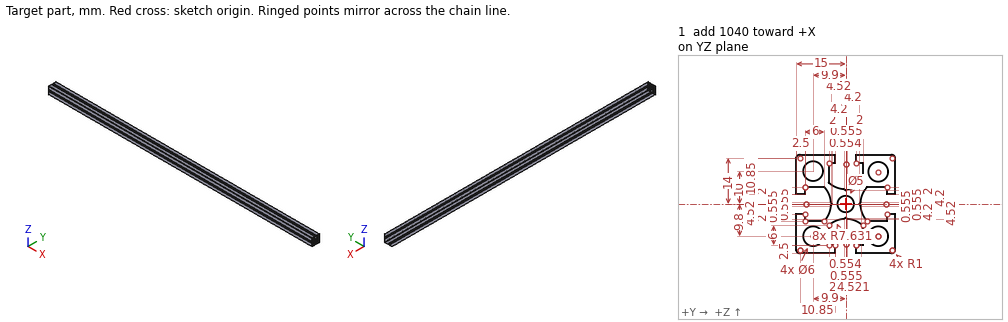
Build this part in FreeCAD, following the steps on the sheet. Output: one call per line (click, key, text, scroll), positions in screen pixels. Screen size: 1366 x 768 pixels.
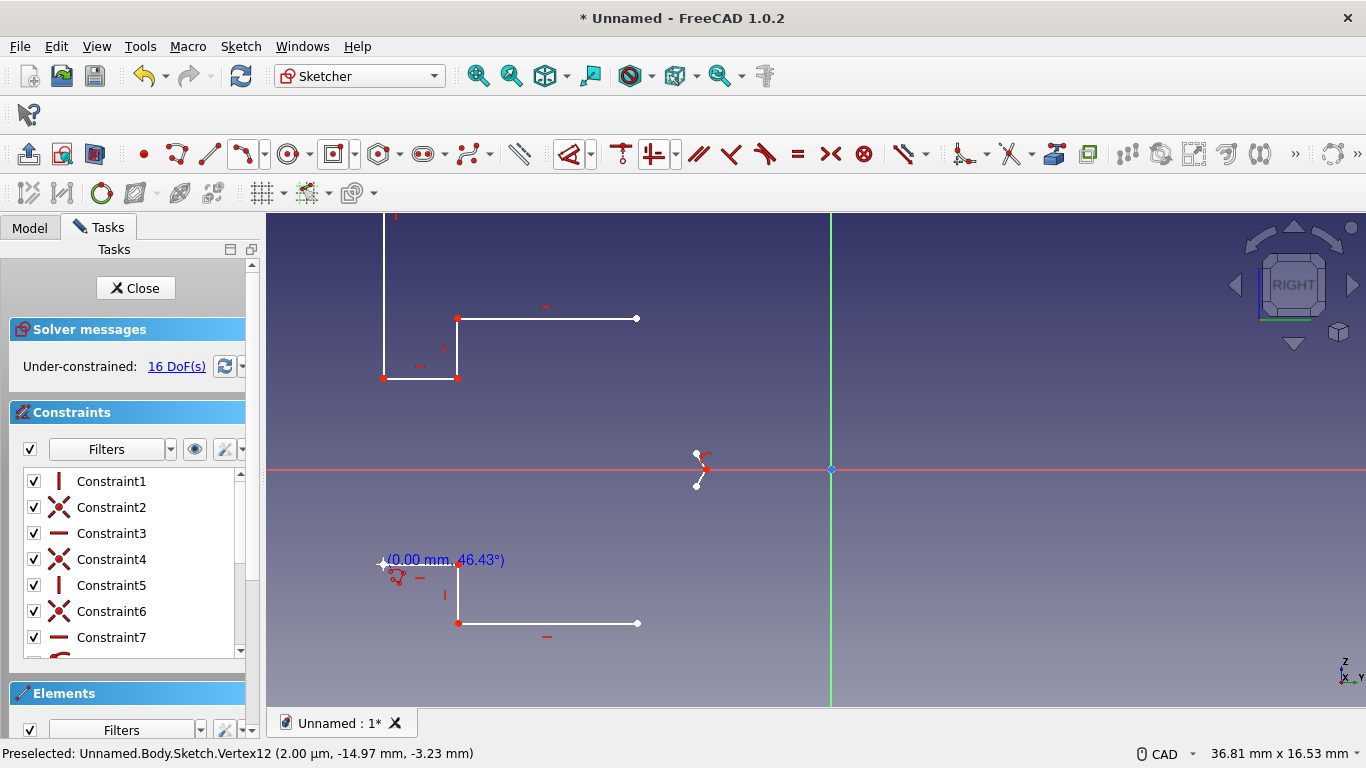
scroll(699, 454, down, 5)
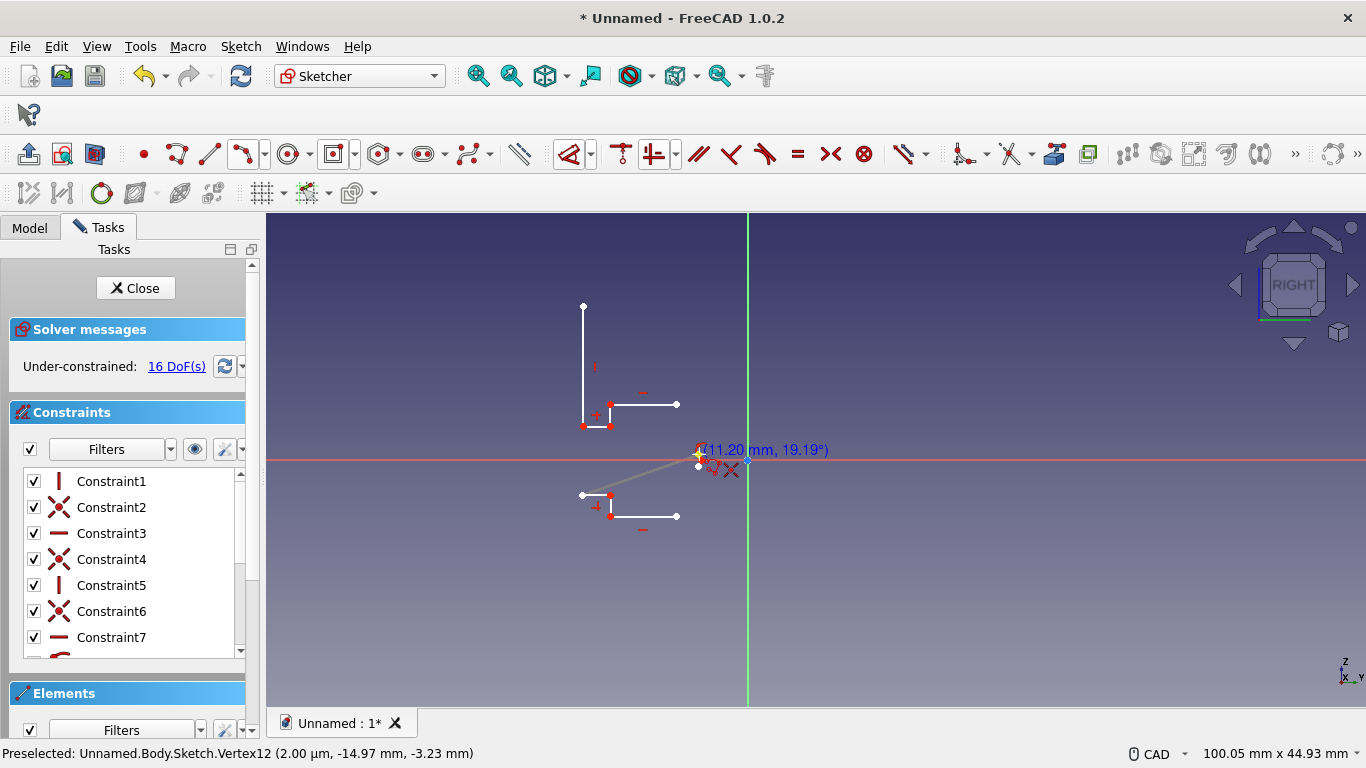
click(583, 614)
right_click(583, 614)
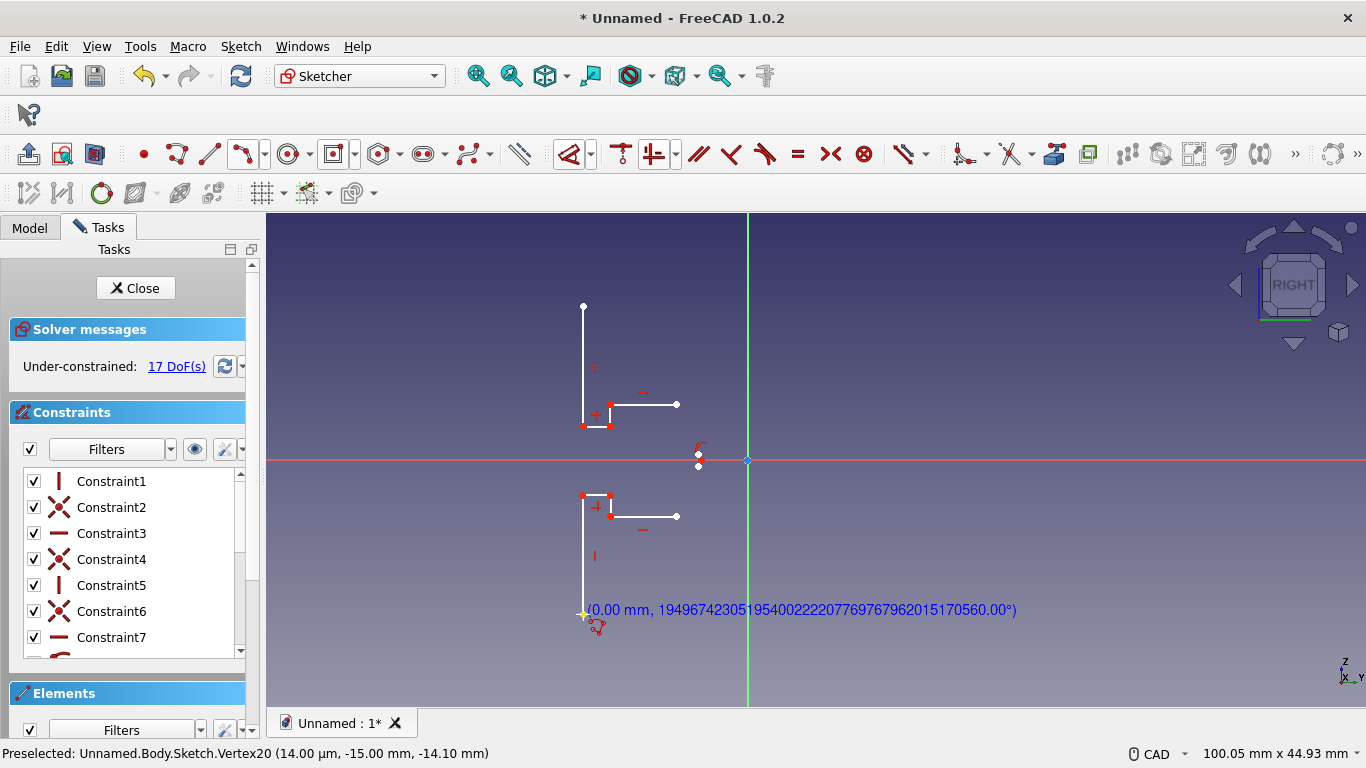
click(594, 625)
click(713, 625)
click(713, 597)
click(691, 597)
click(691, 531)
right_click(691, 531)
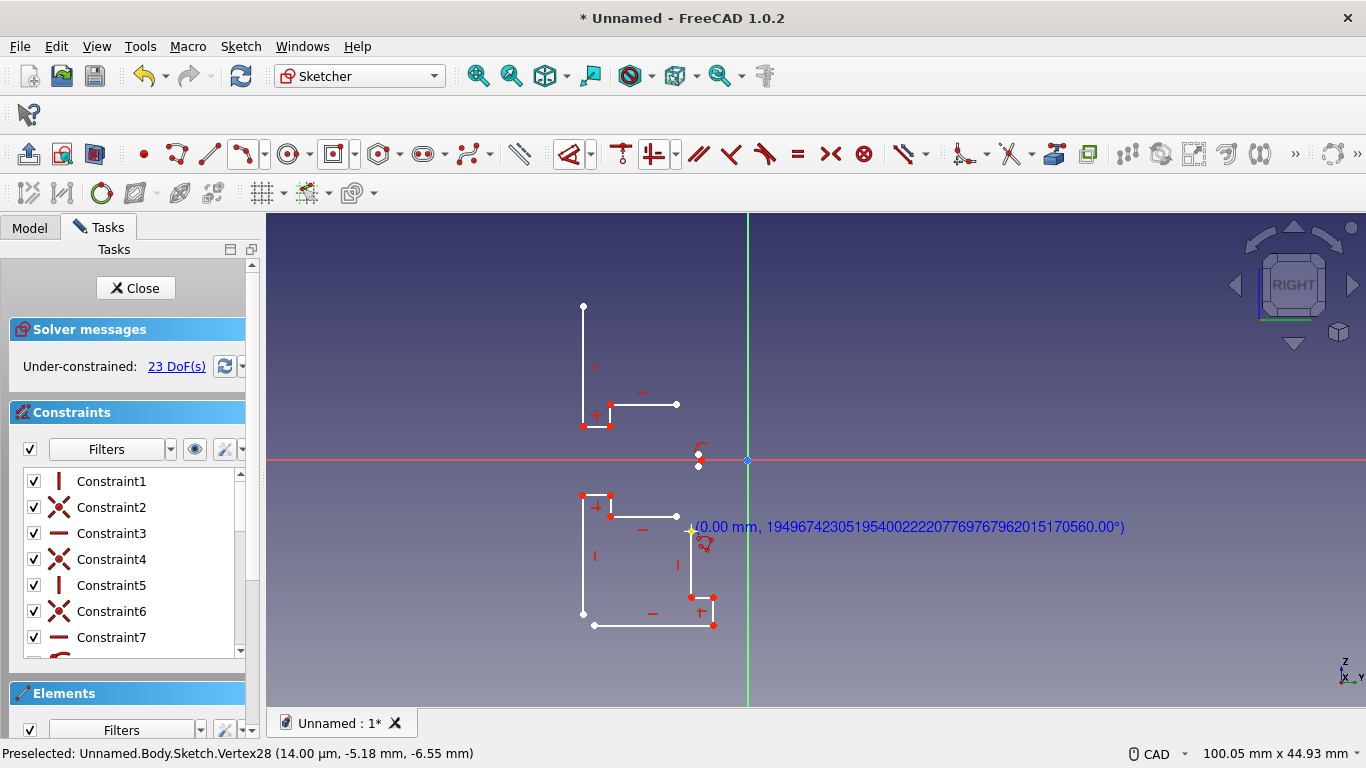
scroll(742, 510, up, 5)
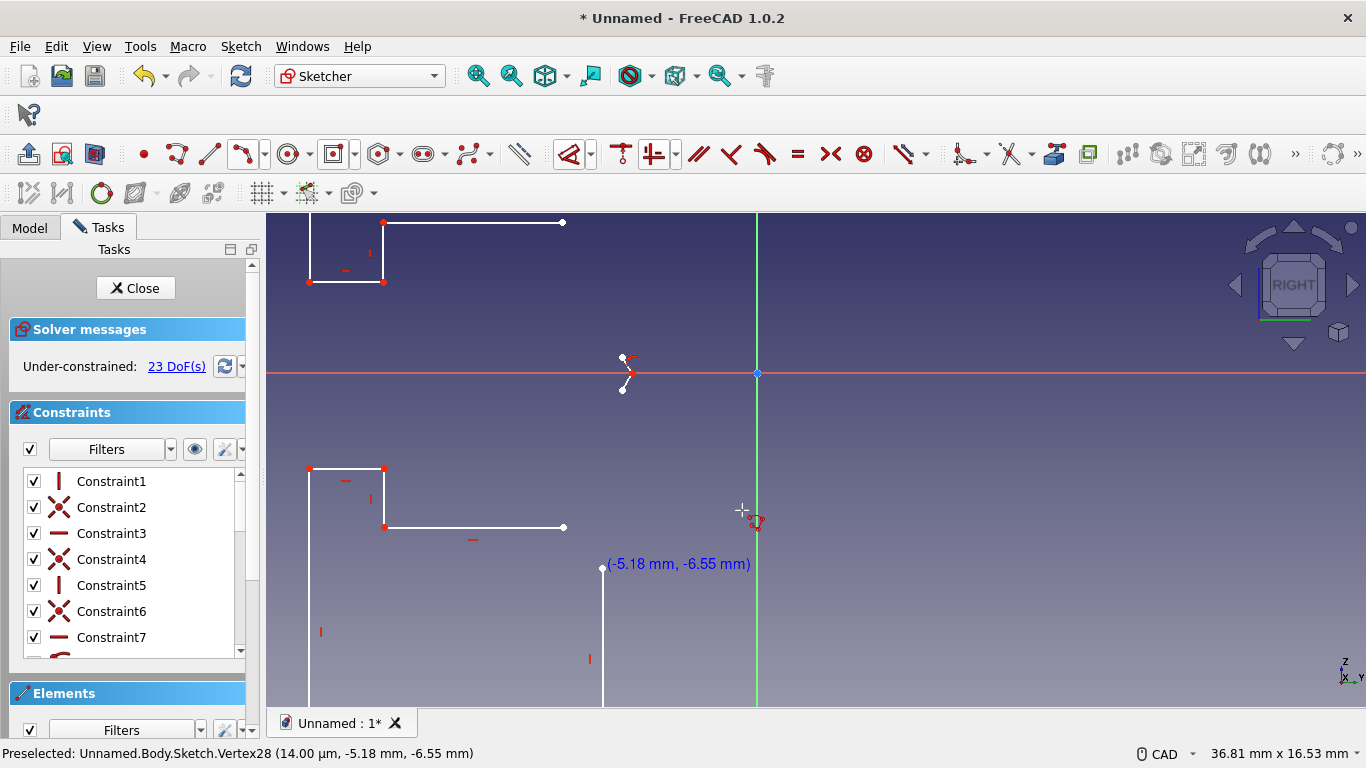
click(741, 508)
click(757, 499)
click(774, 508)
right_click(774, 508)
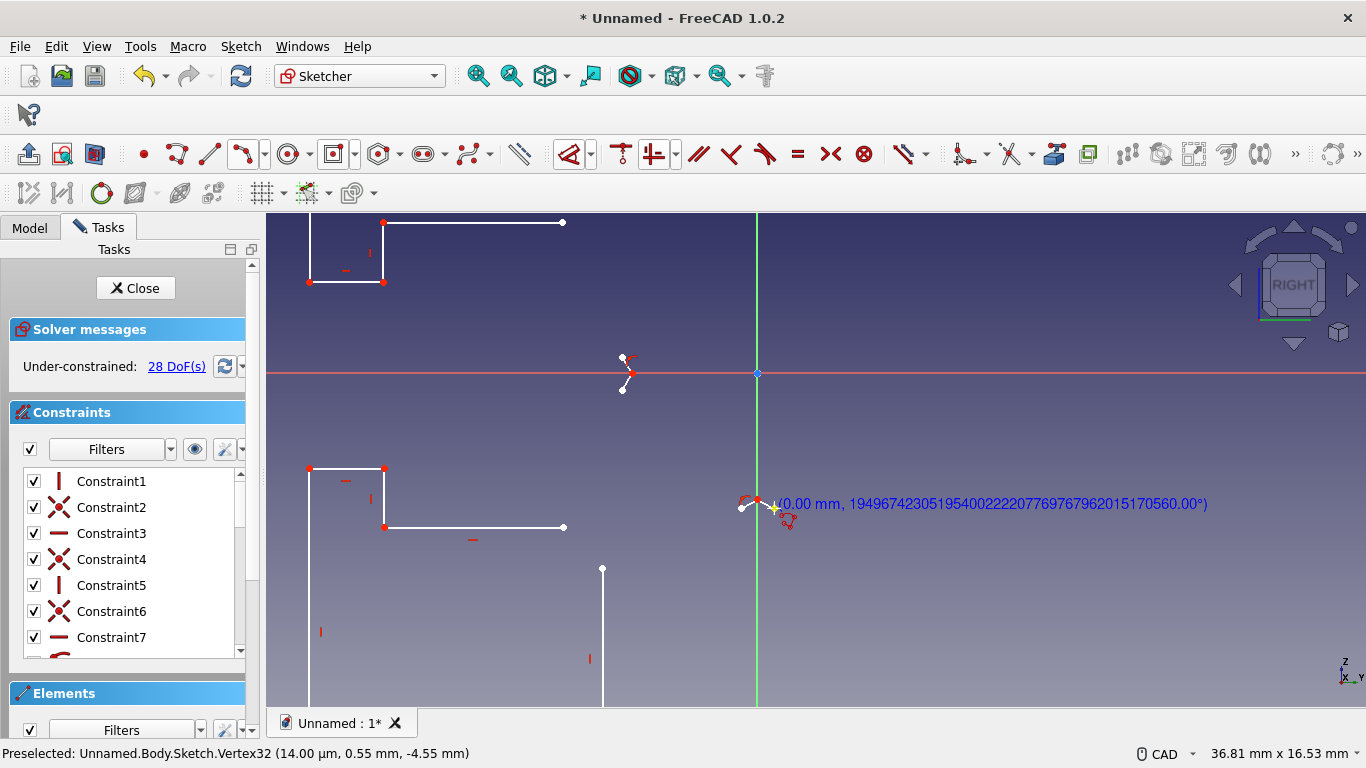
click(911, 567)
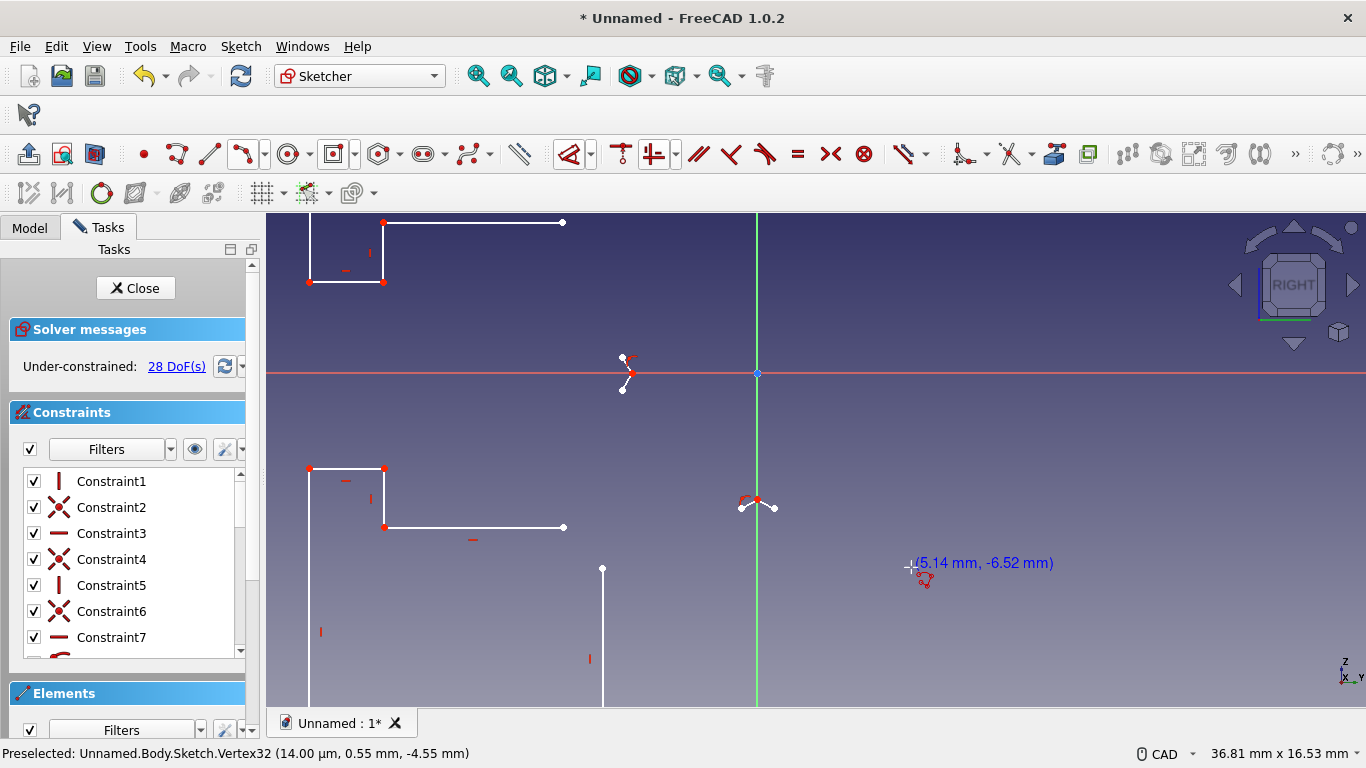
scroll(742, 511, down, 5)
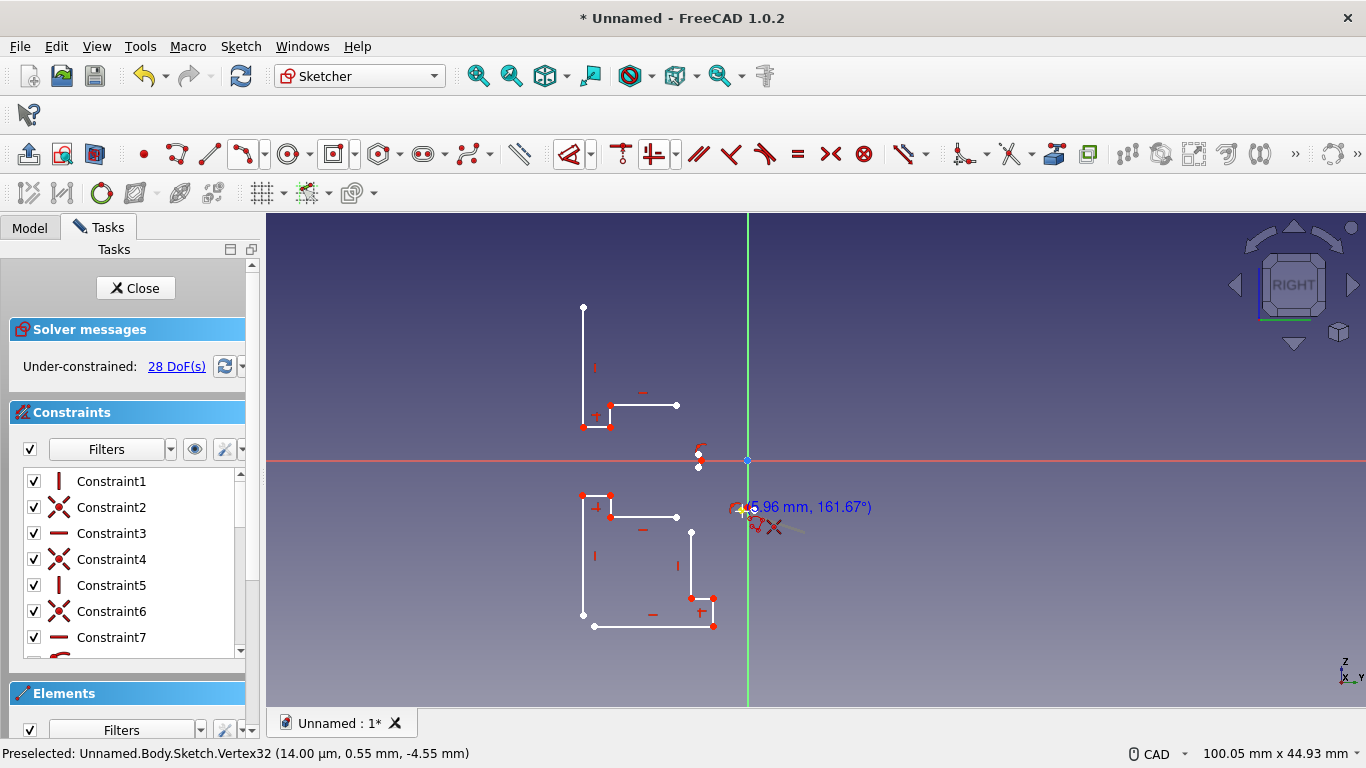
click(804, 598)
click(783, 598)
click(783, 626)
click(902, 626)
right_click(902, 626)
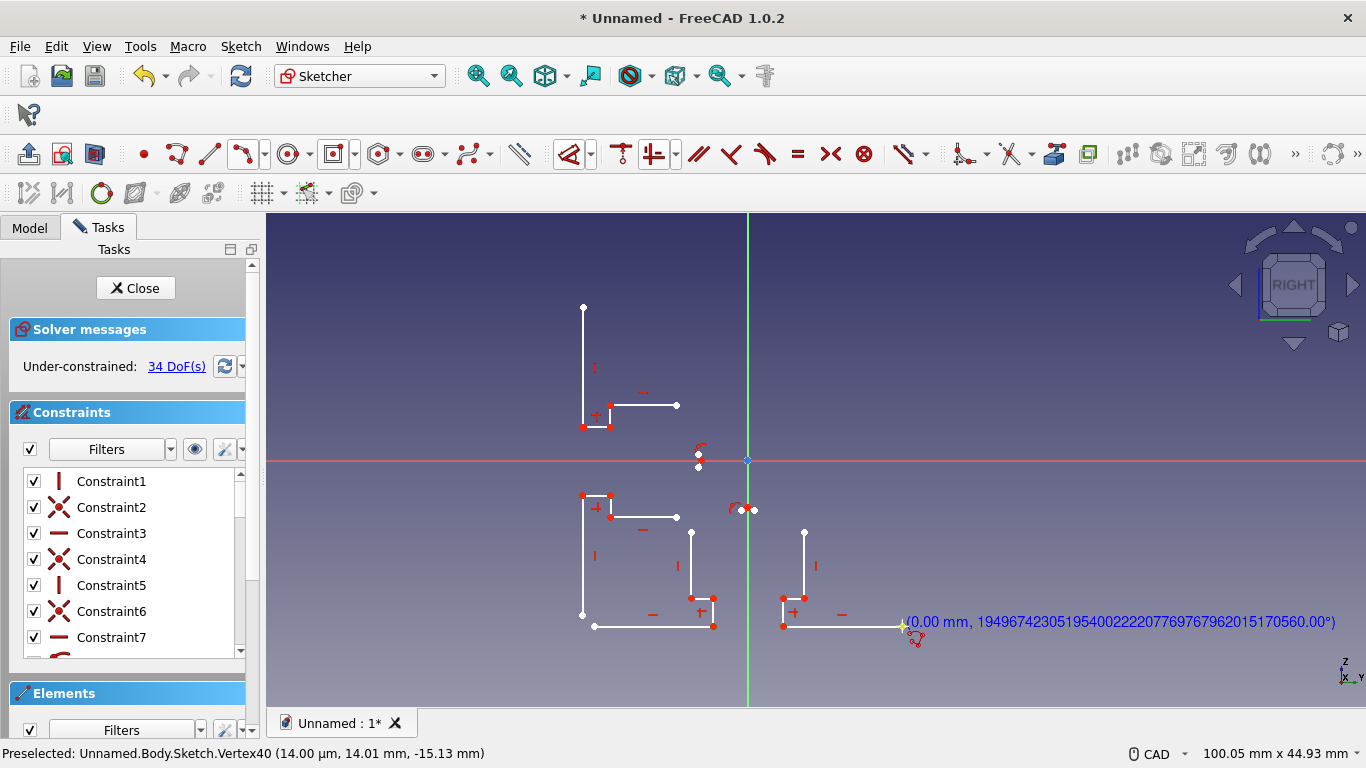
click(913, 615)
click(913, 495)
click(885, 495)
click(885, 517)
click(819, 517)
right_click(819, 517)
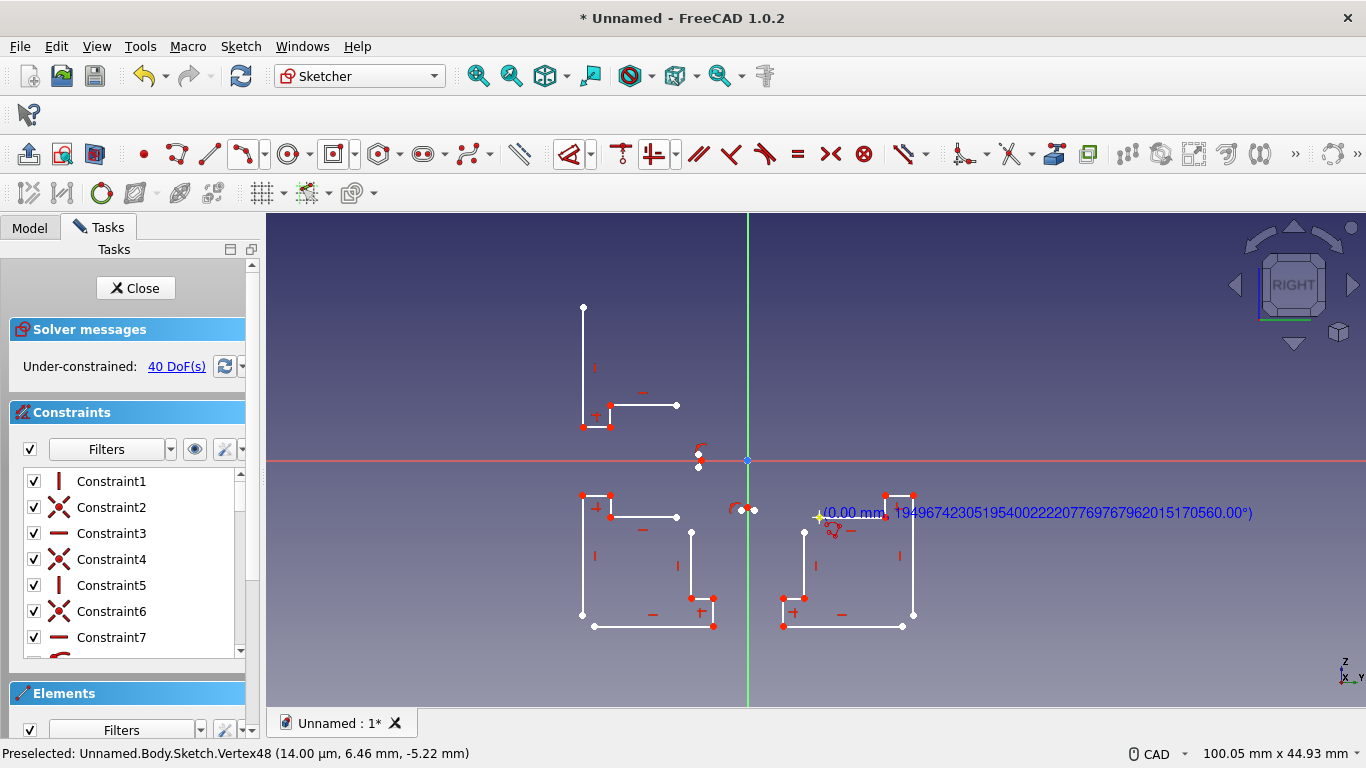
scroll(798, 467, up, 5)